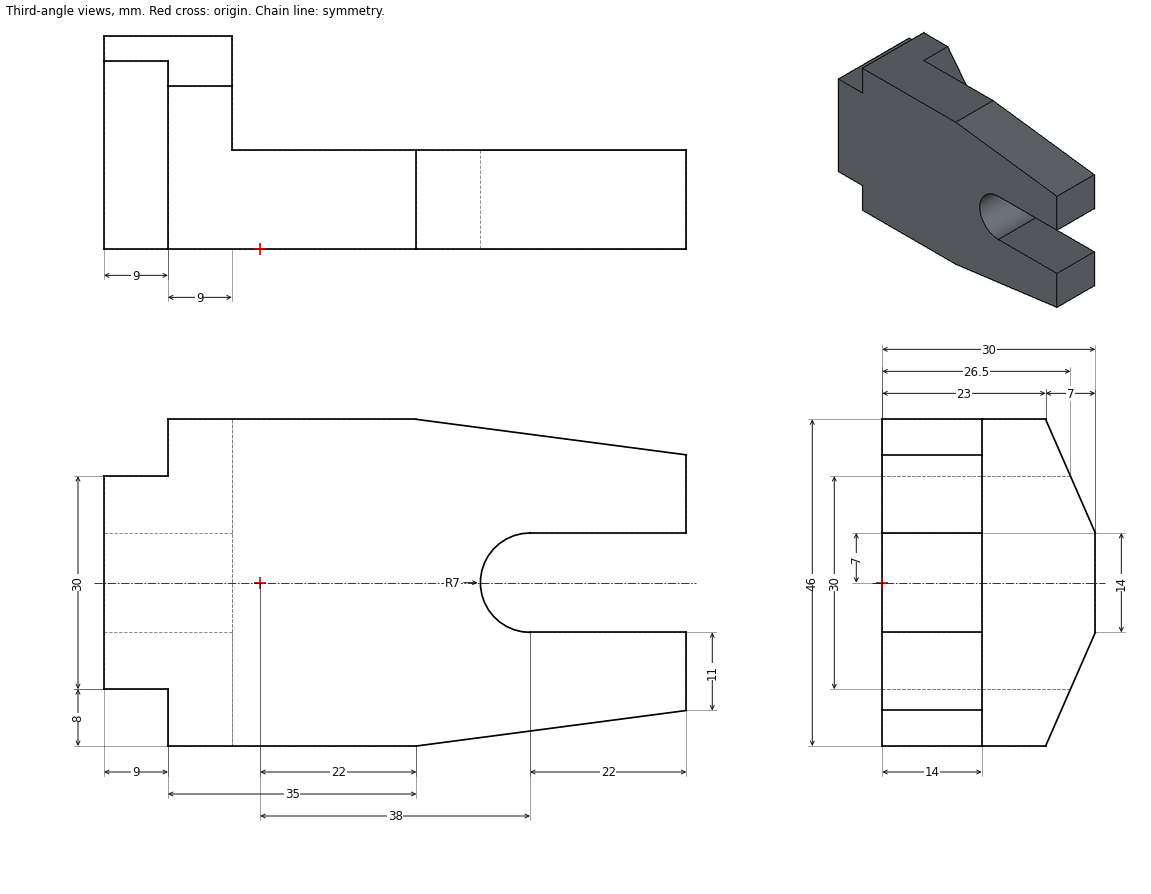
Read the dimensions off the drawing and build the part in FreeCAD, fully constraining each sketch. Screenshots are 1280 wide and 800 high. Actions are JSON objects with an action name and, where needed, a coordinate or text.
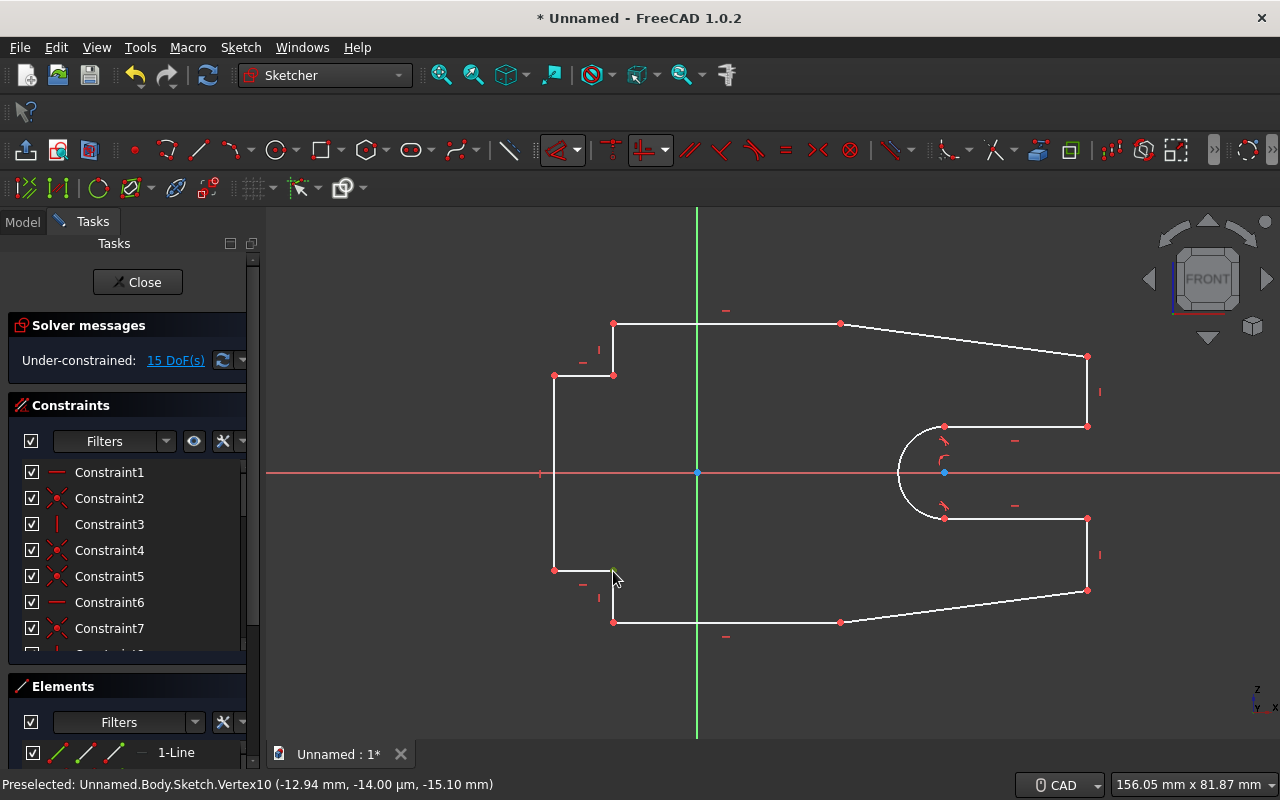
{"action": "left_click", "coordinate": [613, 376]}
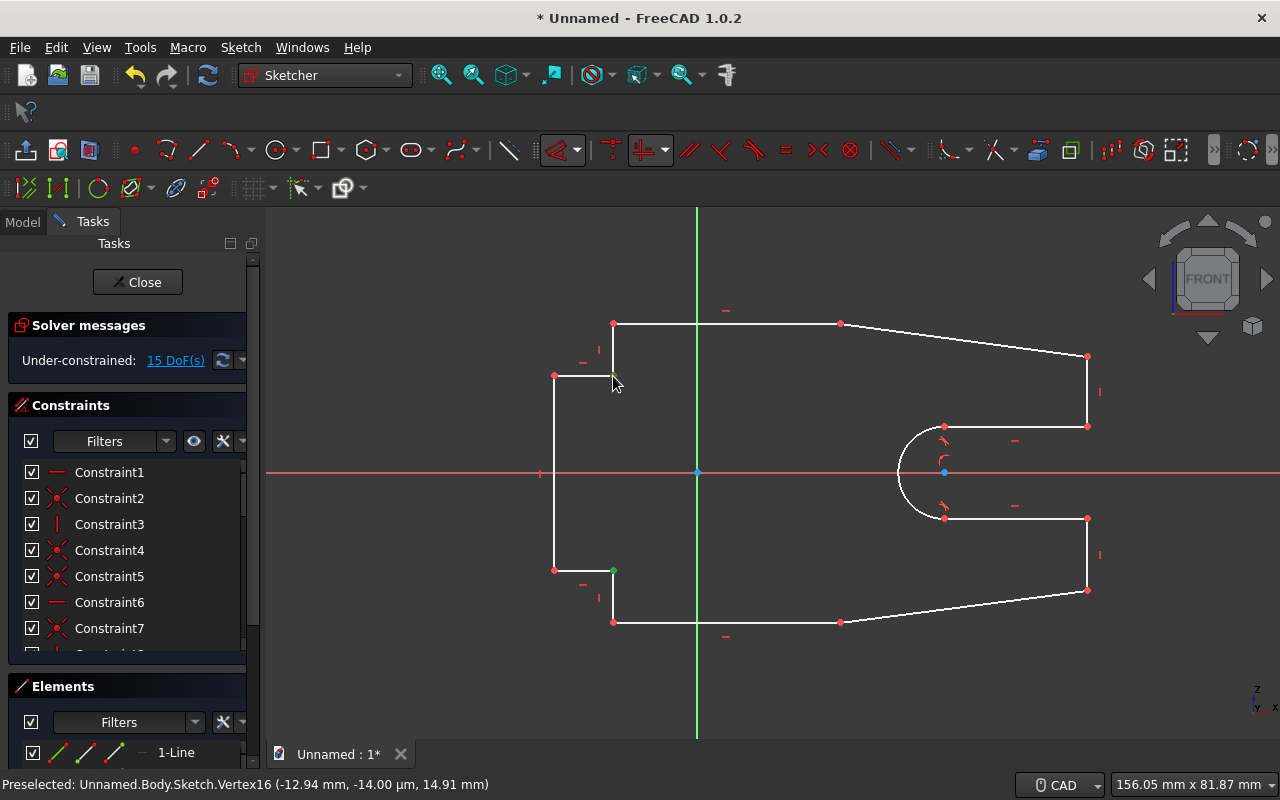
{"action": "left_click", "coordinate": [353, 473]}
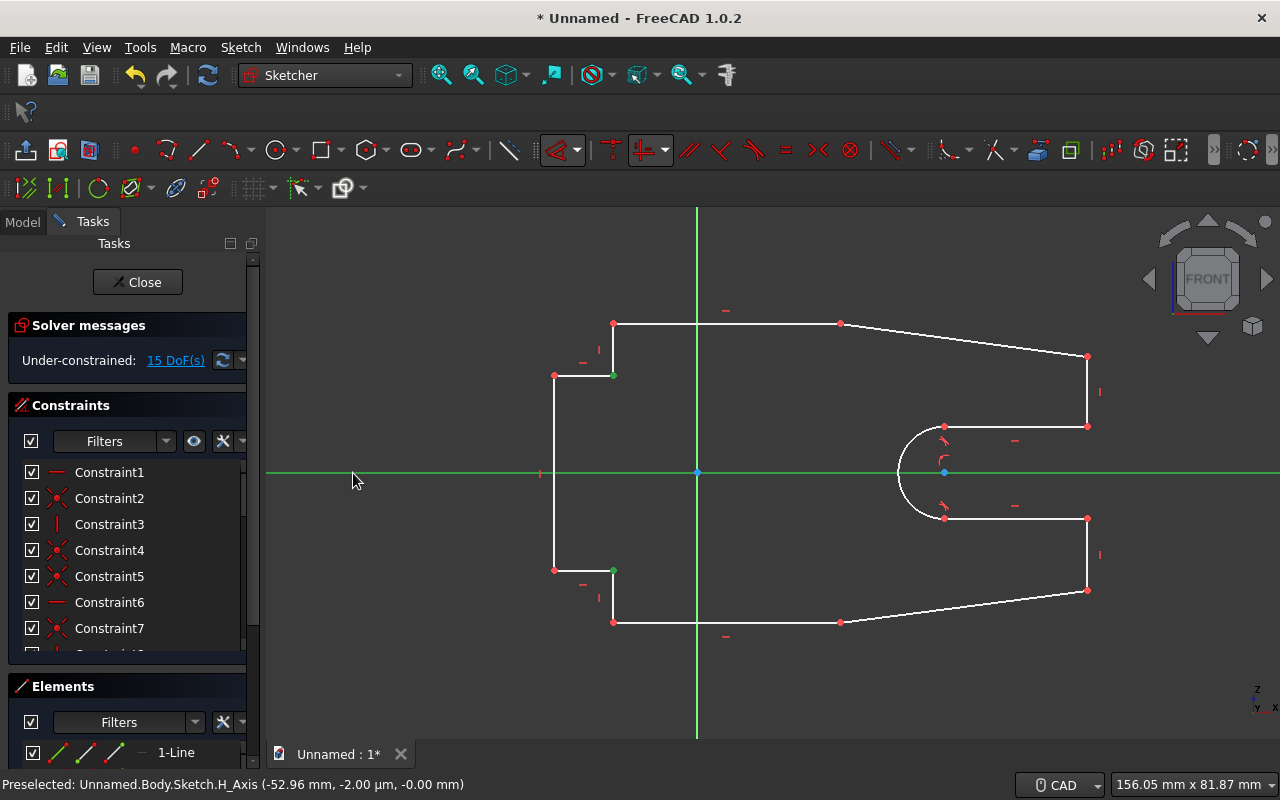
{"action": "key", "text": "s"}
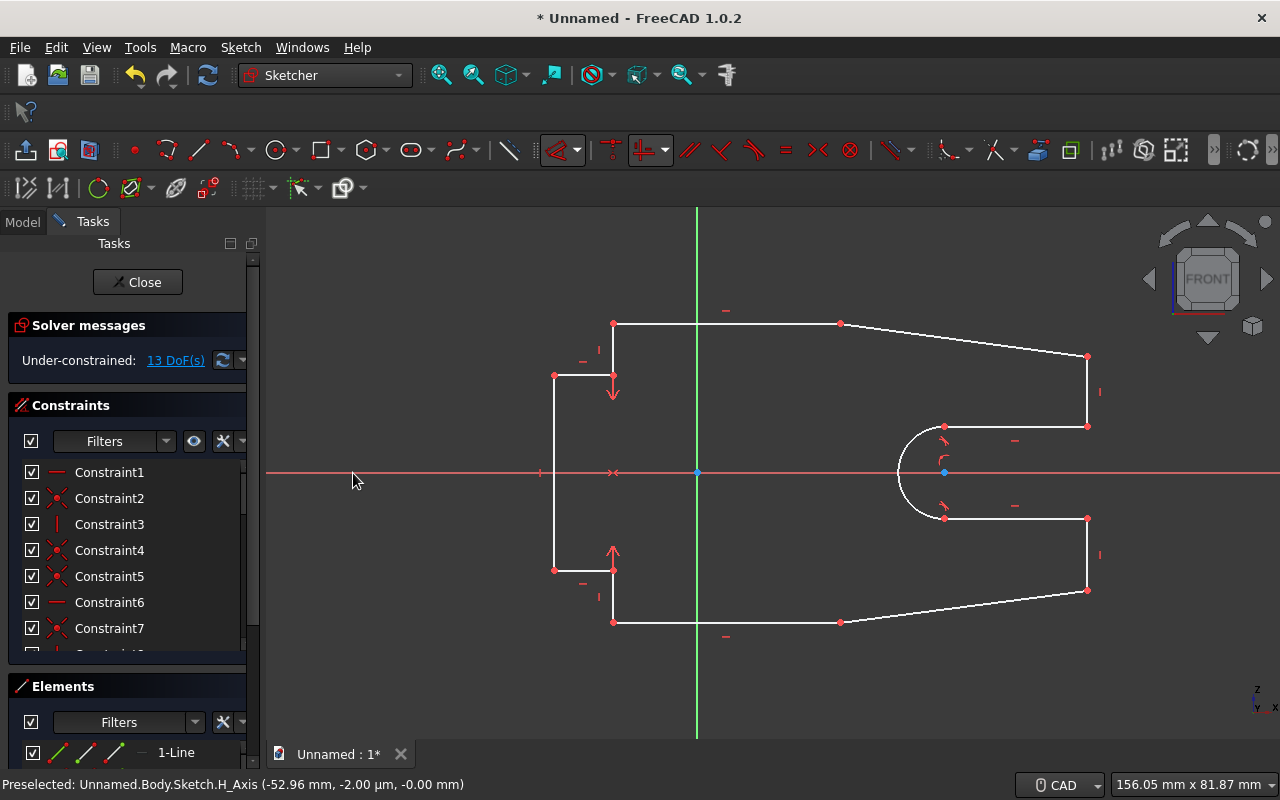
{"action": "left_click", "coordinate": [840, 623]}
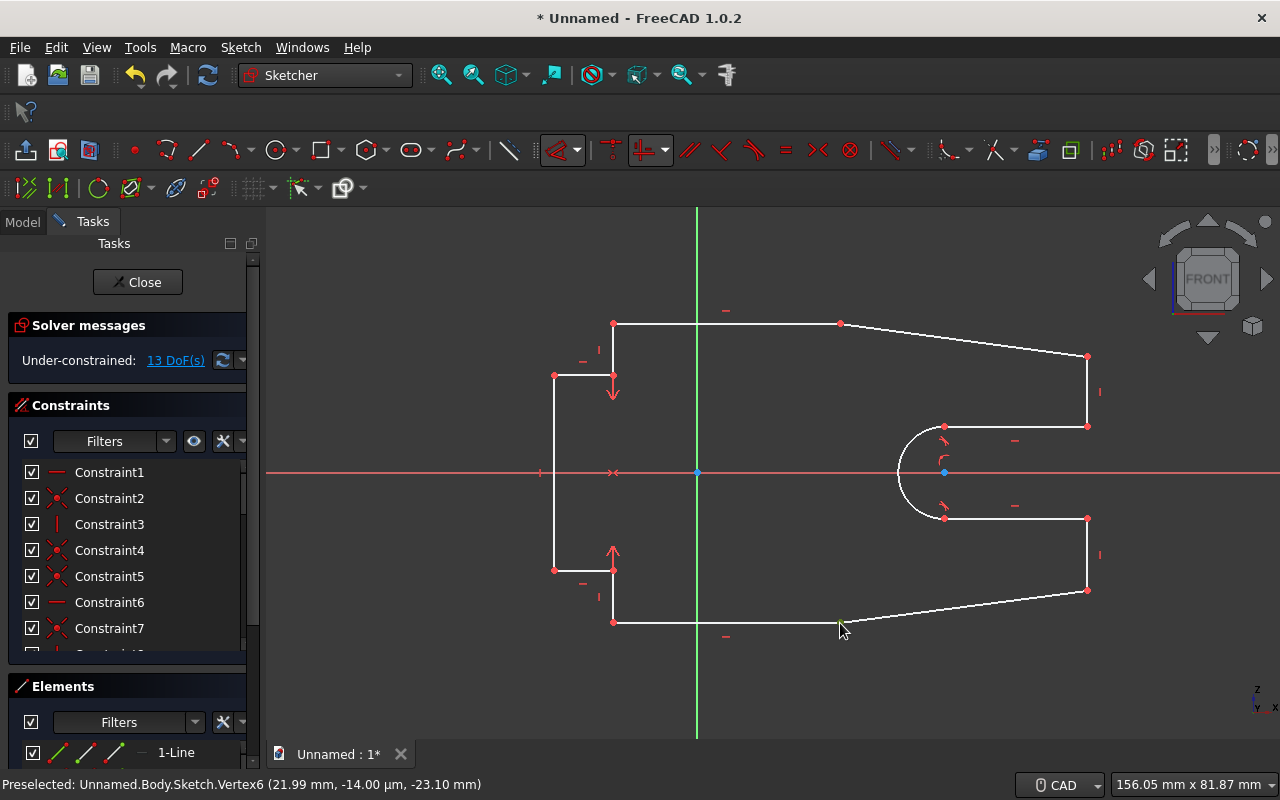
{"action": "left_click", "coordinate": [840, 324]}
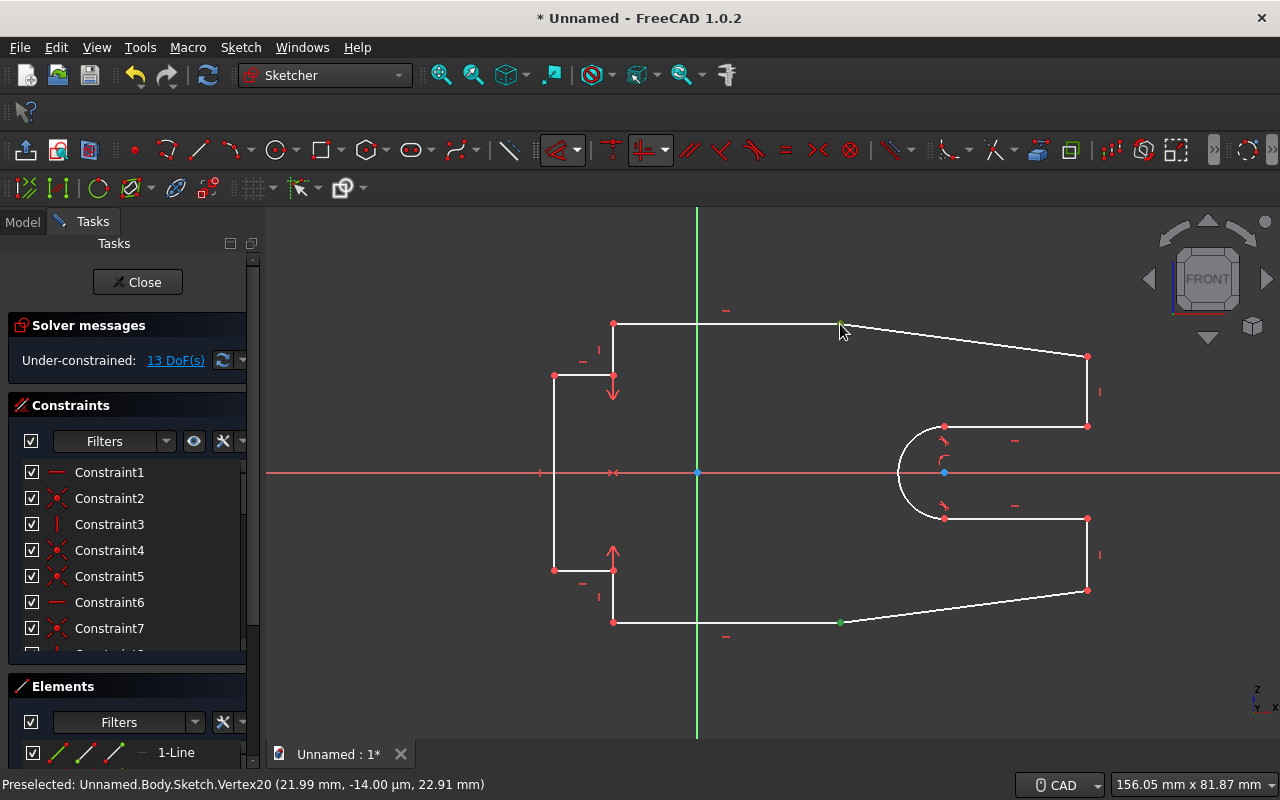
{"action": "left_click", "coordinate": [353, 473]}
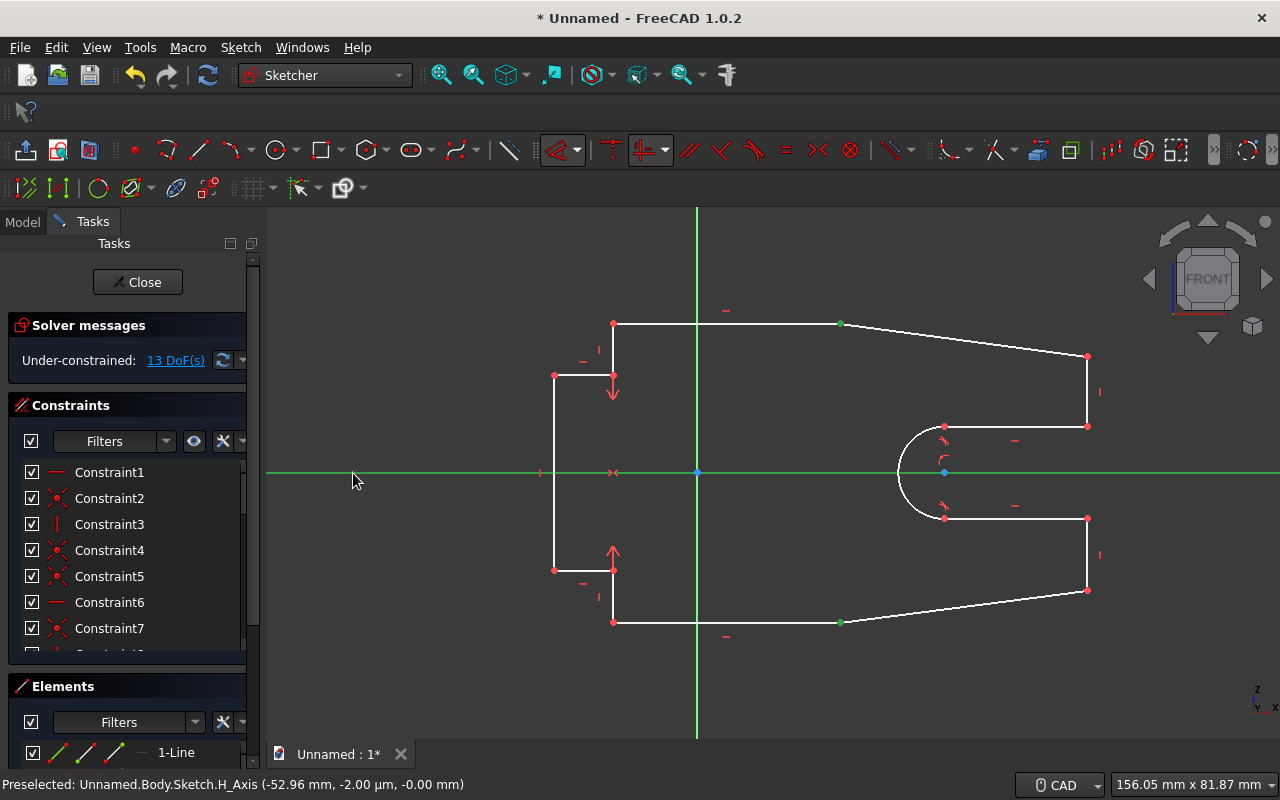
{"action": "key", "text": "s"}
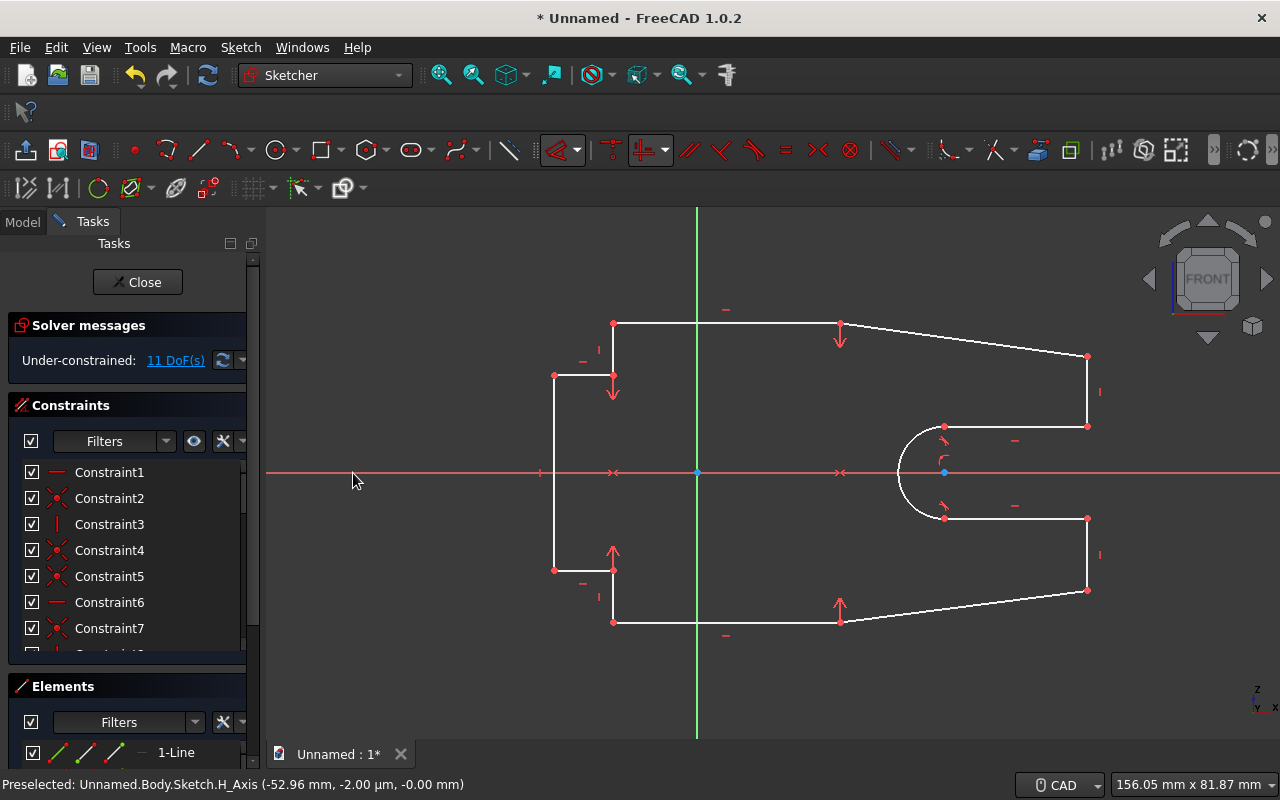
{"action": "left_click", "coordinate": [1087, 591]}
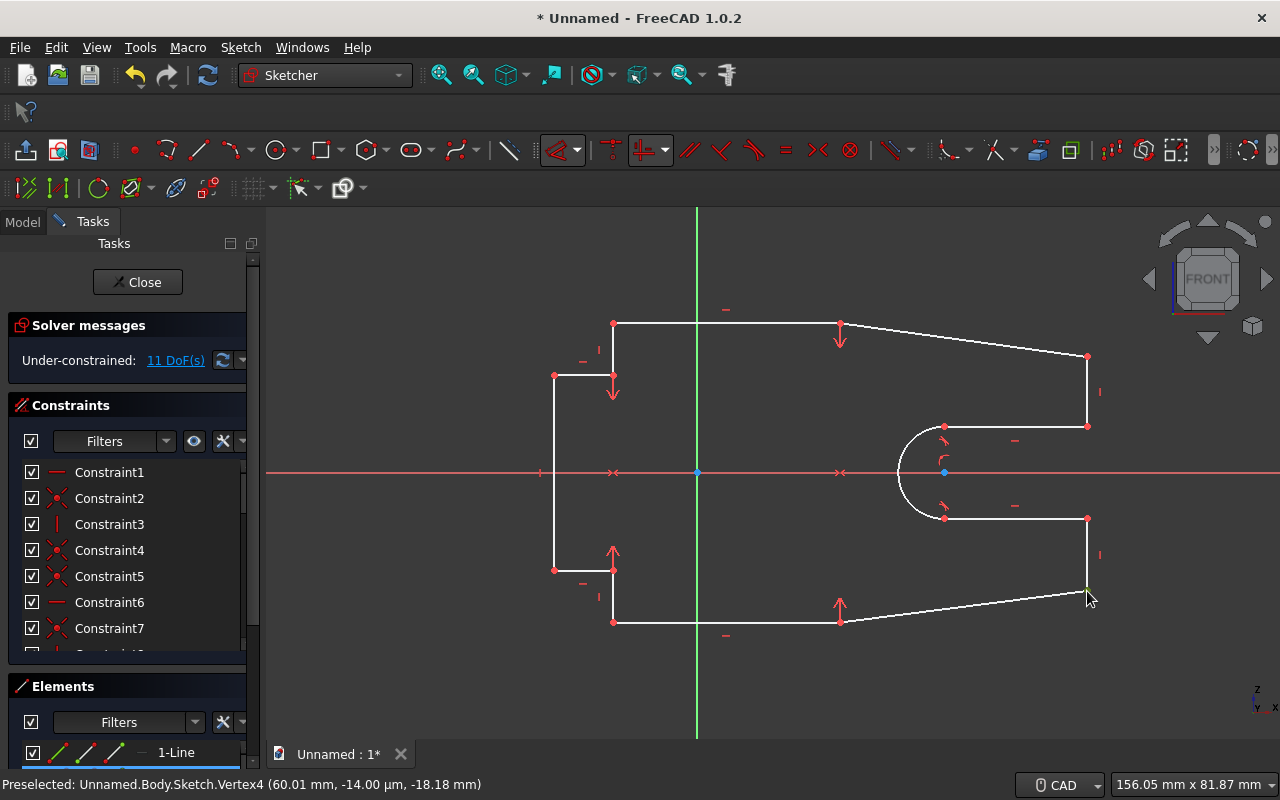
{"action": "left_click", "coordinate": [1087, 357]}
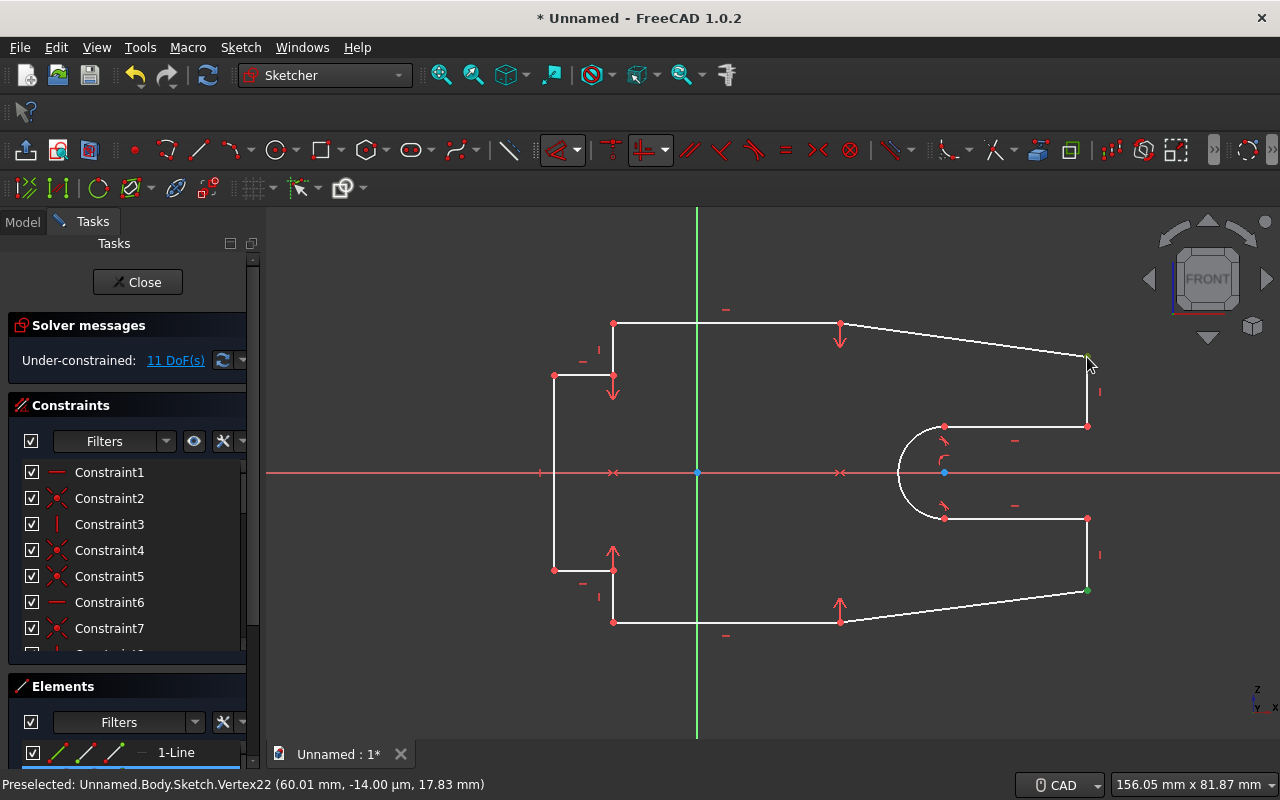
{"action": "left_click", "coordinate": [353, 473]}